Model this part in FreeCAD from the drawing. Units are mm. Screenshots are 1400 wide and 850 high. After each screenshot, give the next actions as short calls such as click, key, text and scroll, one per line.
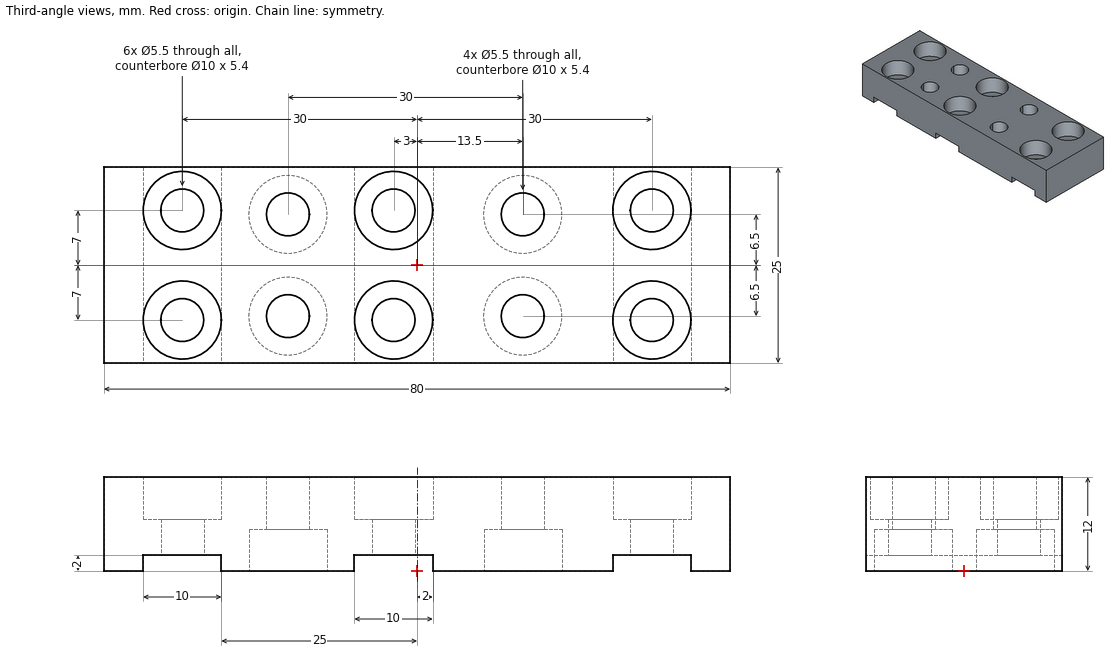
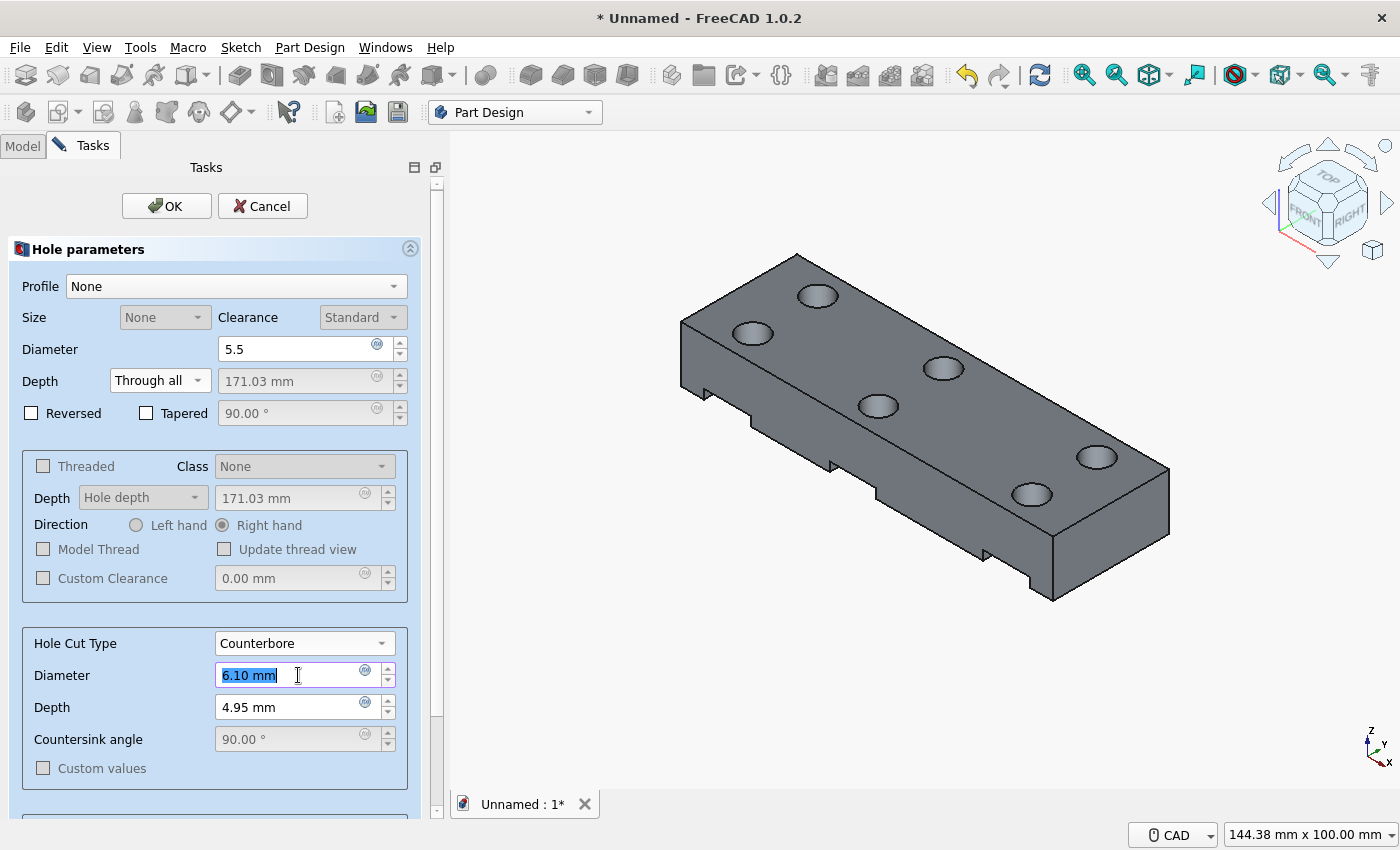
text(10)
key(Tab)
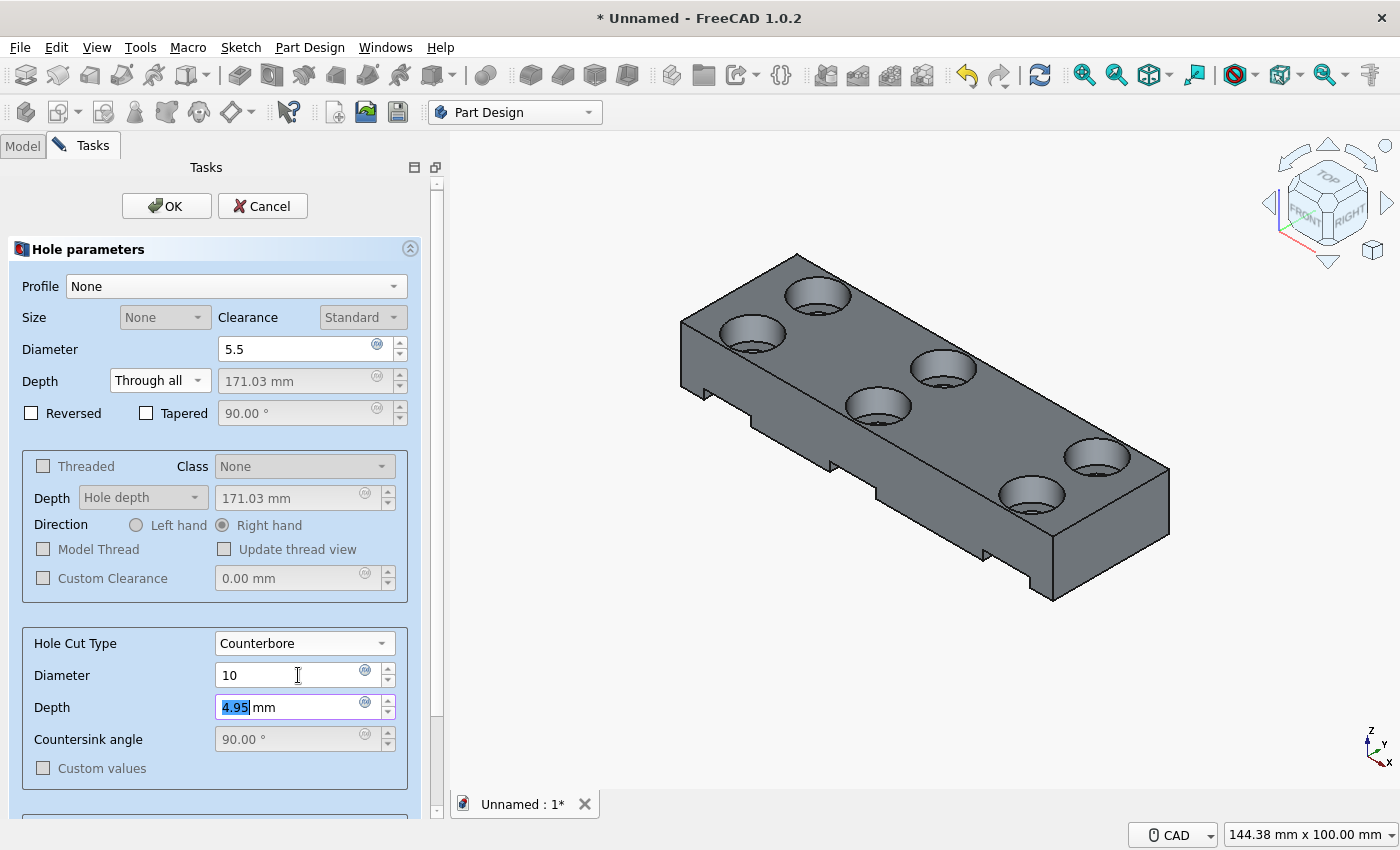
text(5.4)
key(Tab)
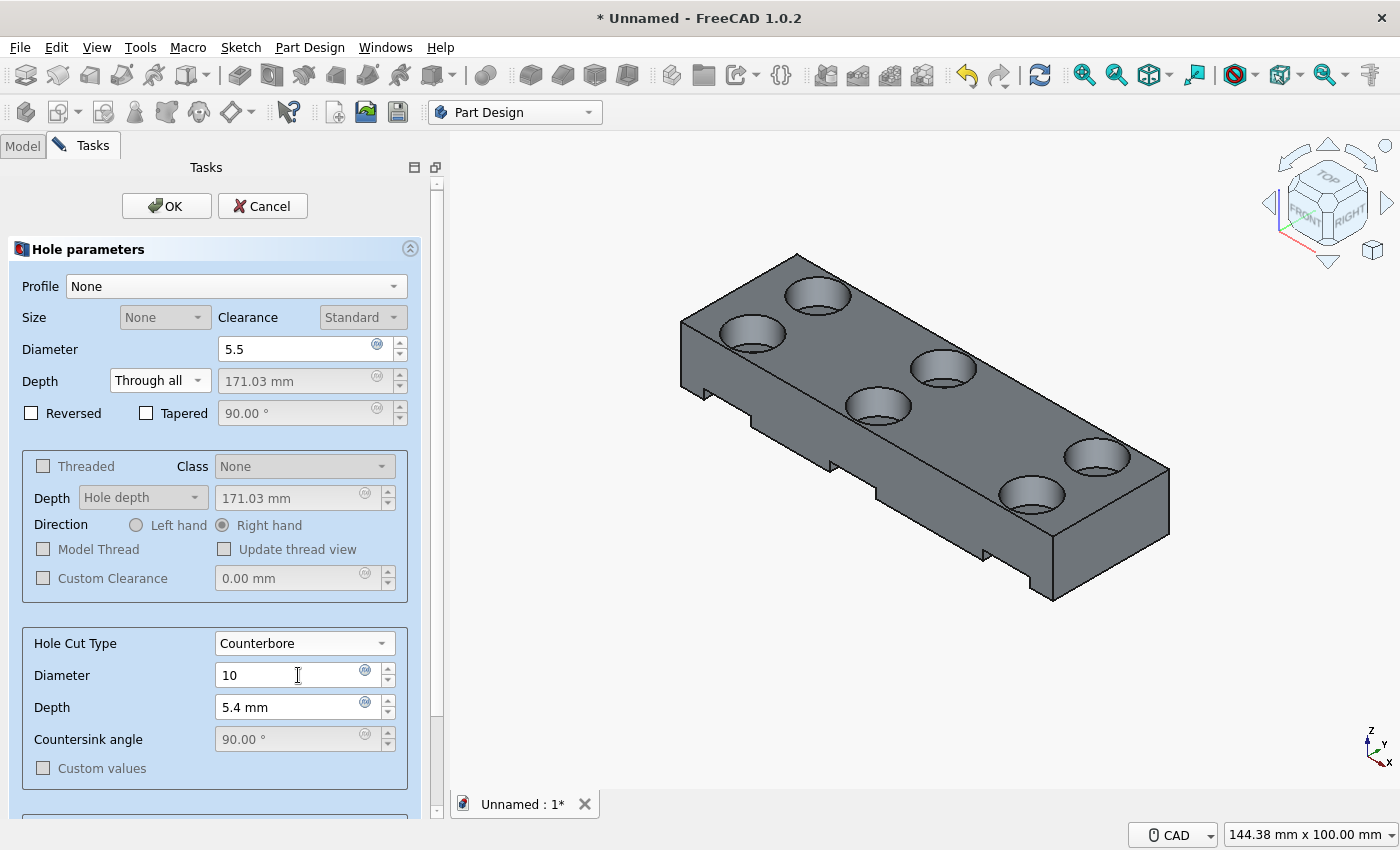
click(167, 206)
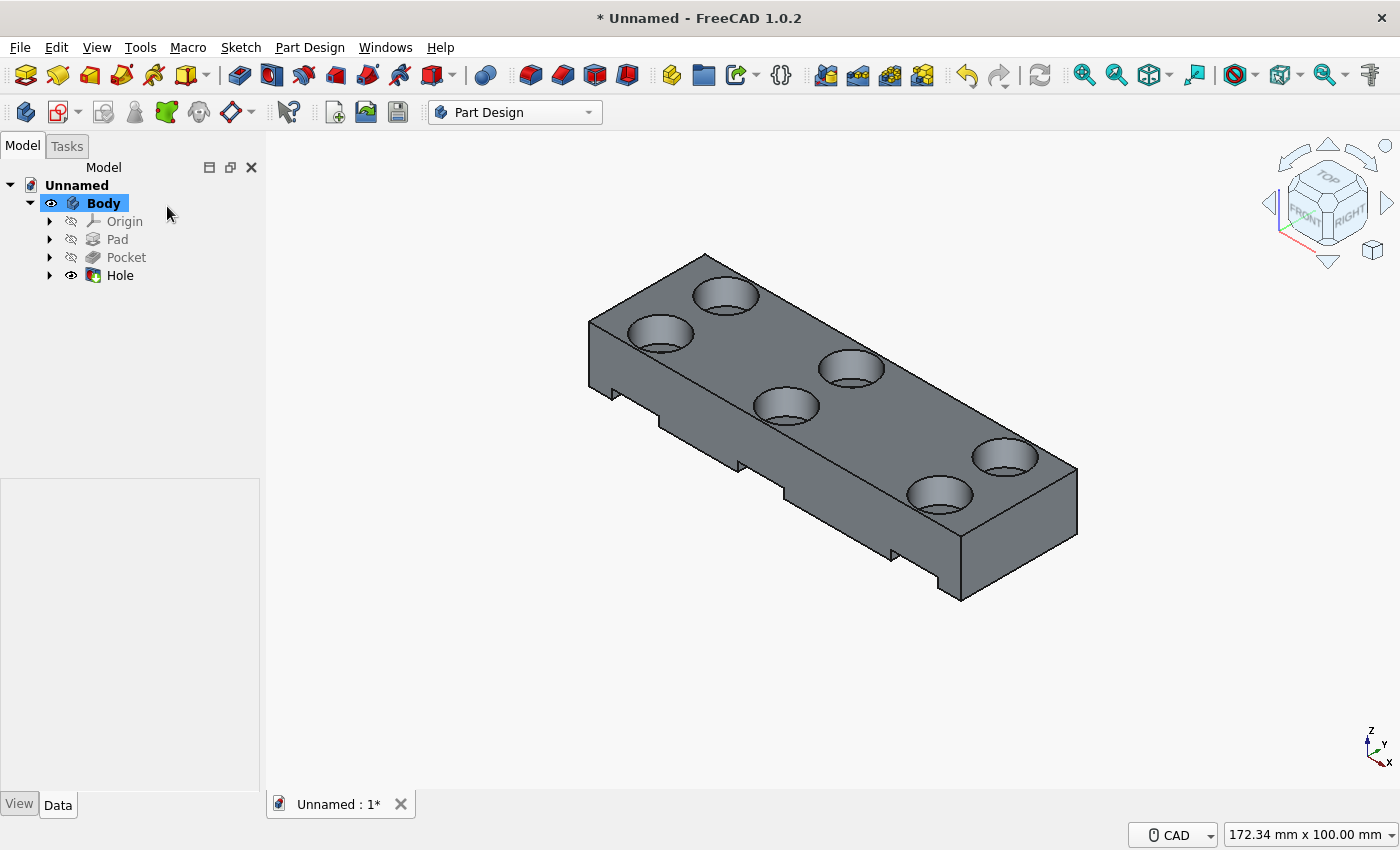
key(5)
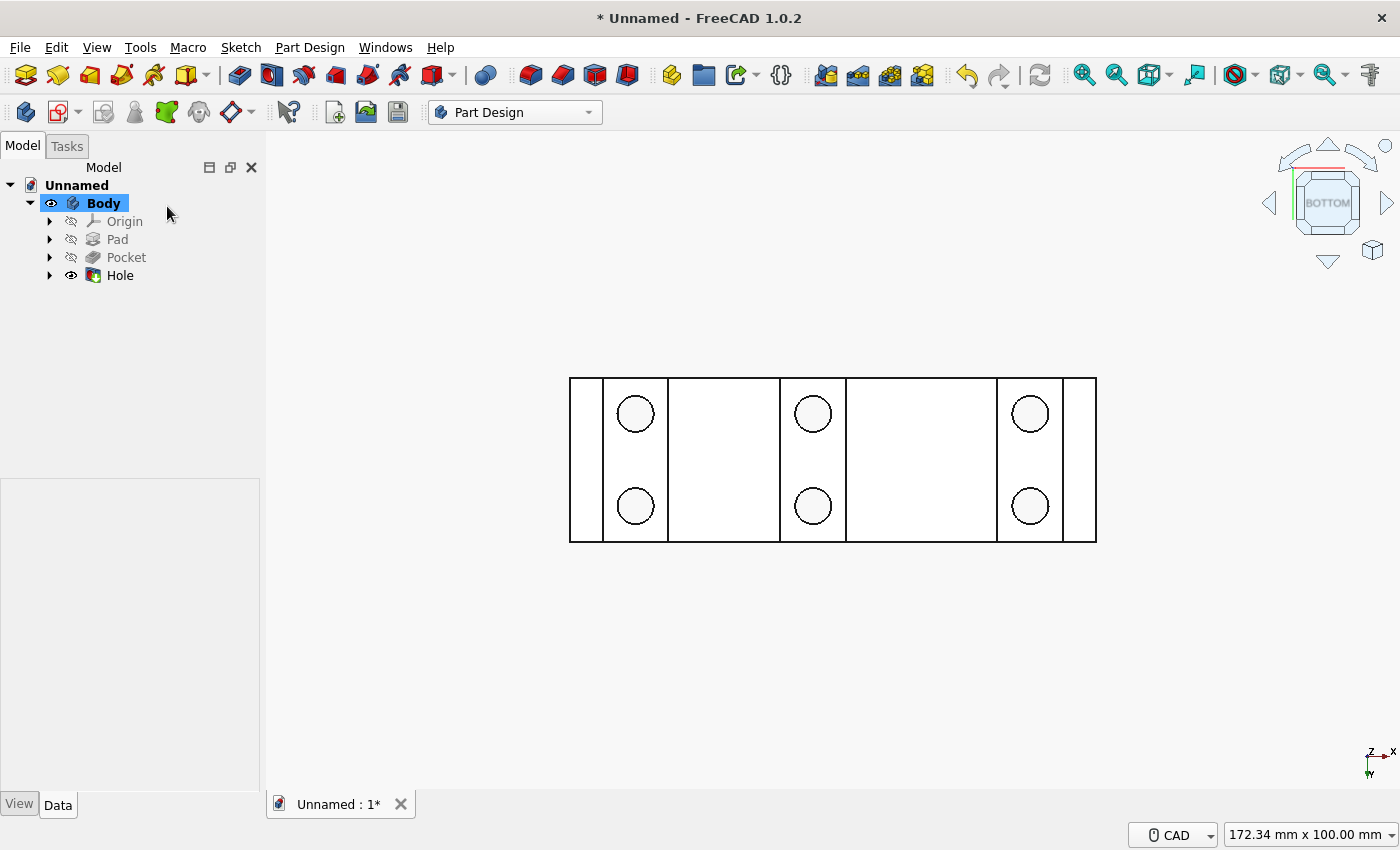
click(922, 459)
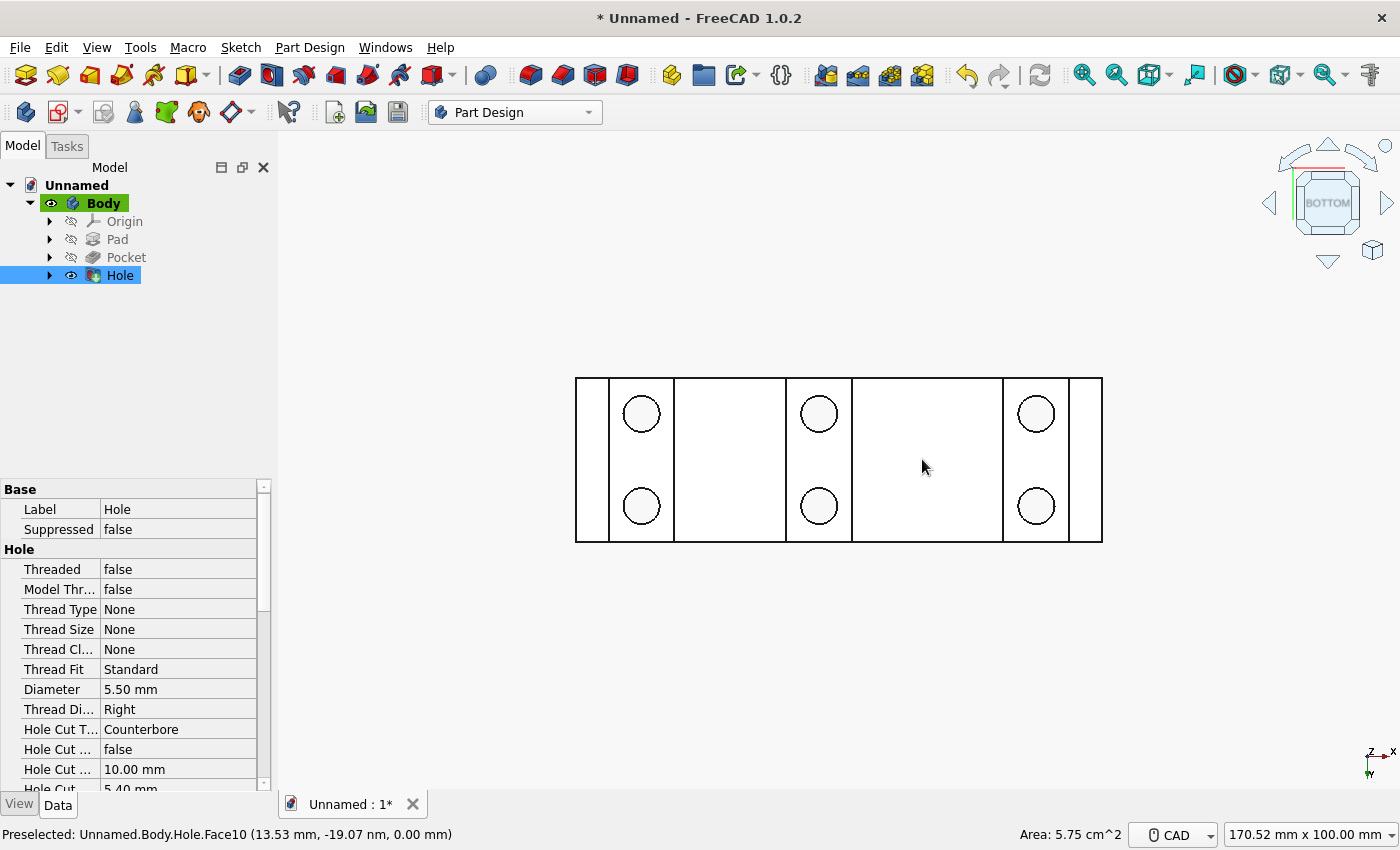
click(58, 112)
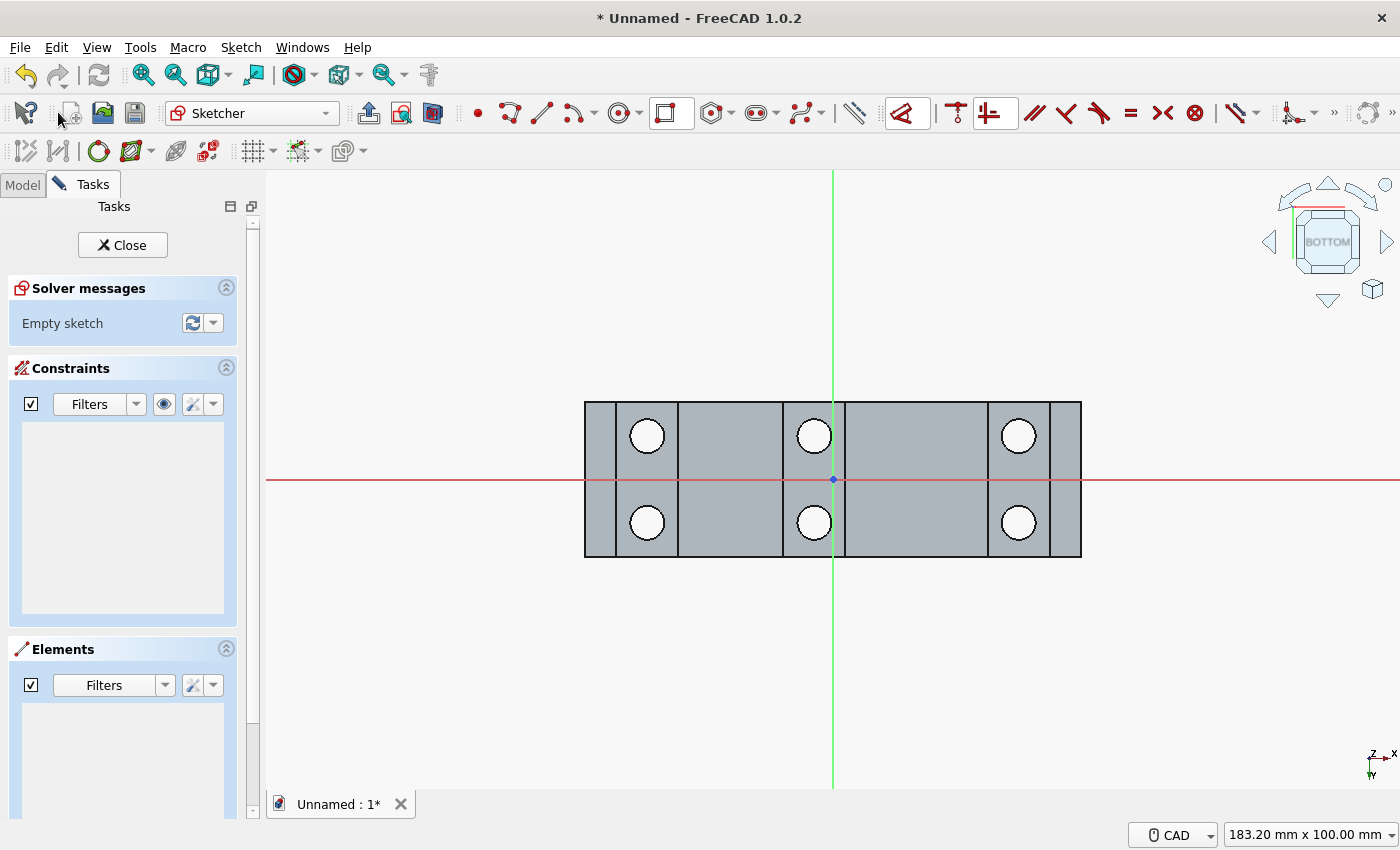
scroll(849, 480, up, 6)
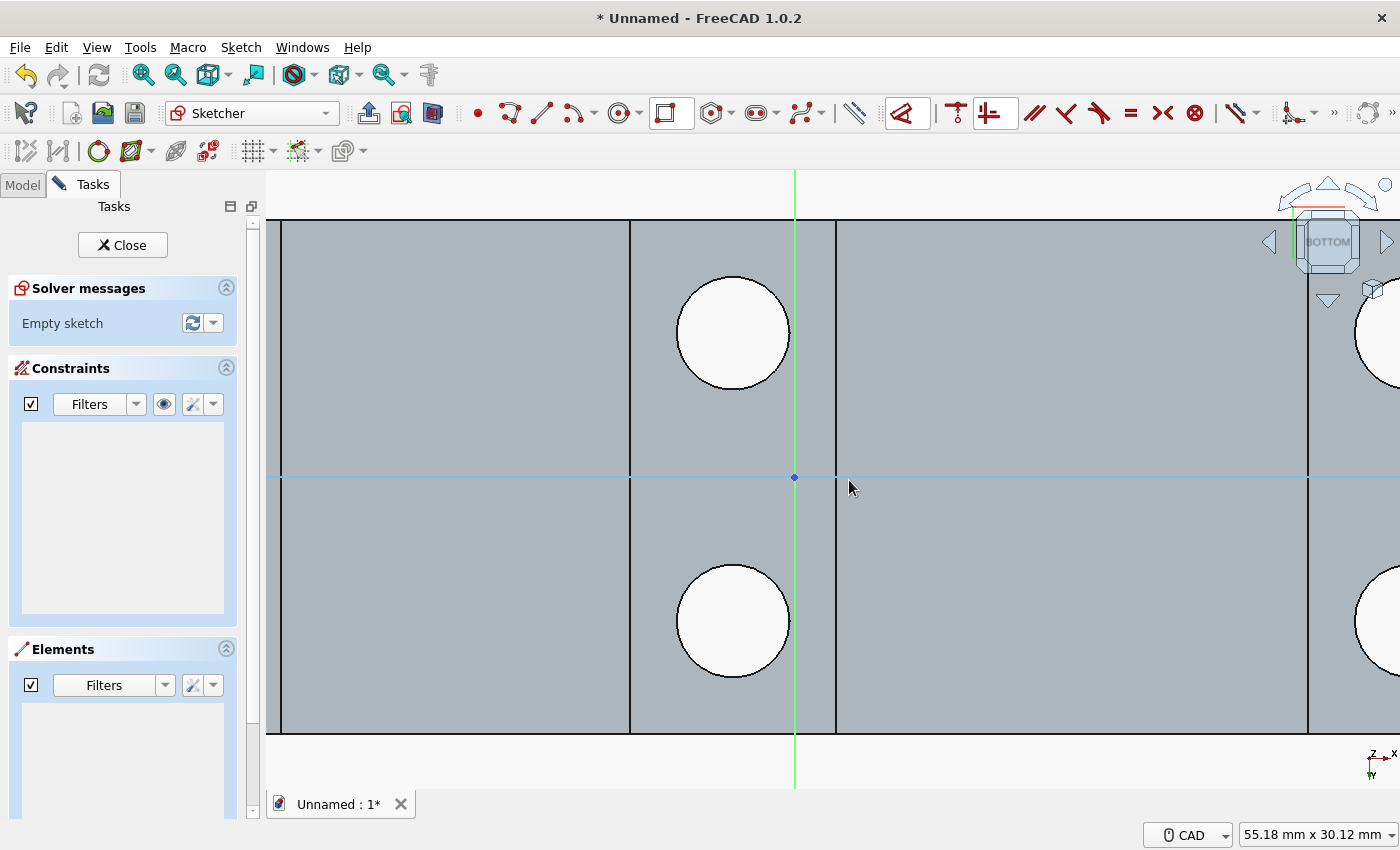
click(620, 114)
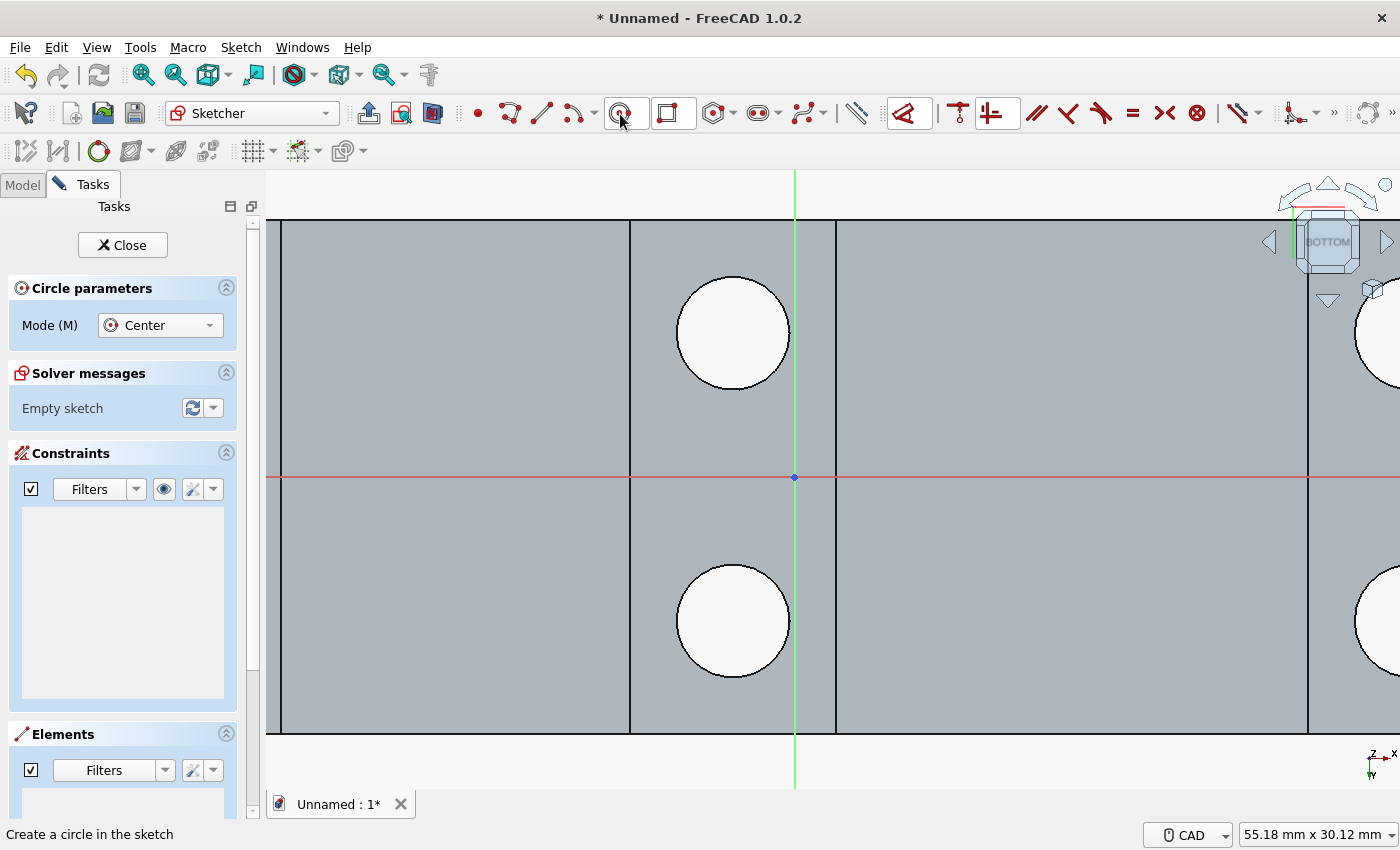
click(1072, 611)
click(1112, 571)